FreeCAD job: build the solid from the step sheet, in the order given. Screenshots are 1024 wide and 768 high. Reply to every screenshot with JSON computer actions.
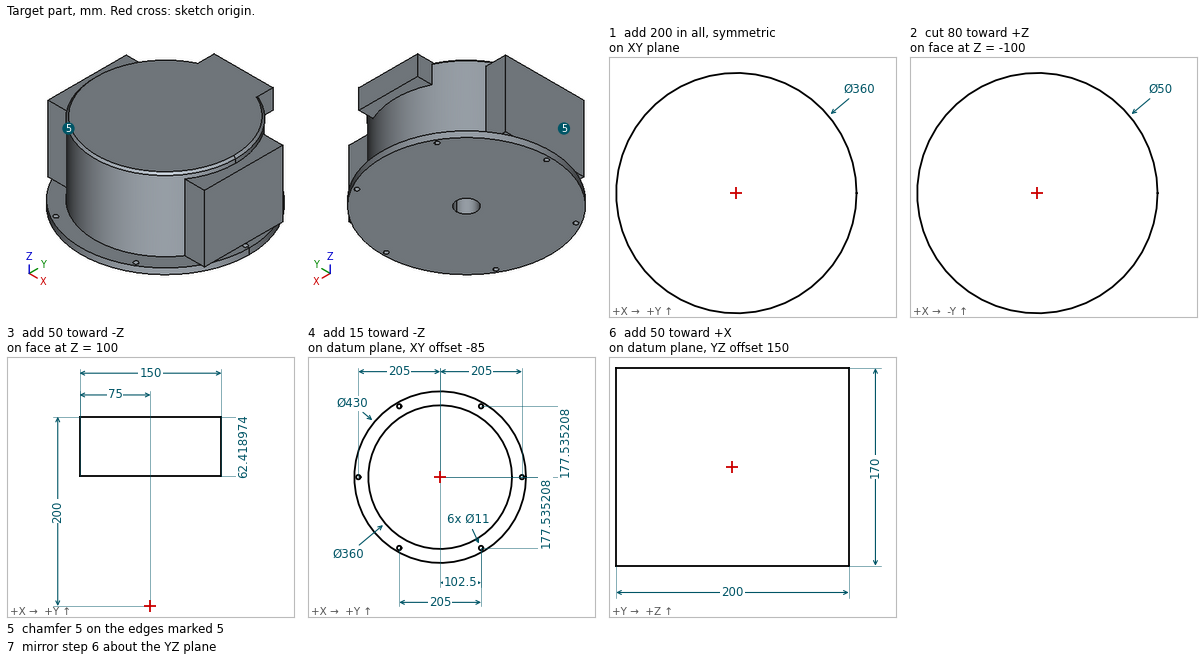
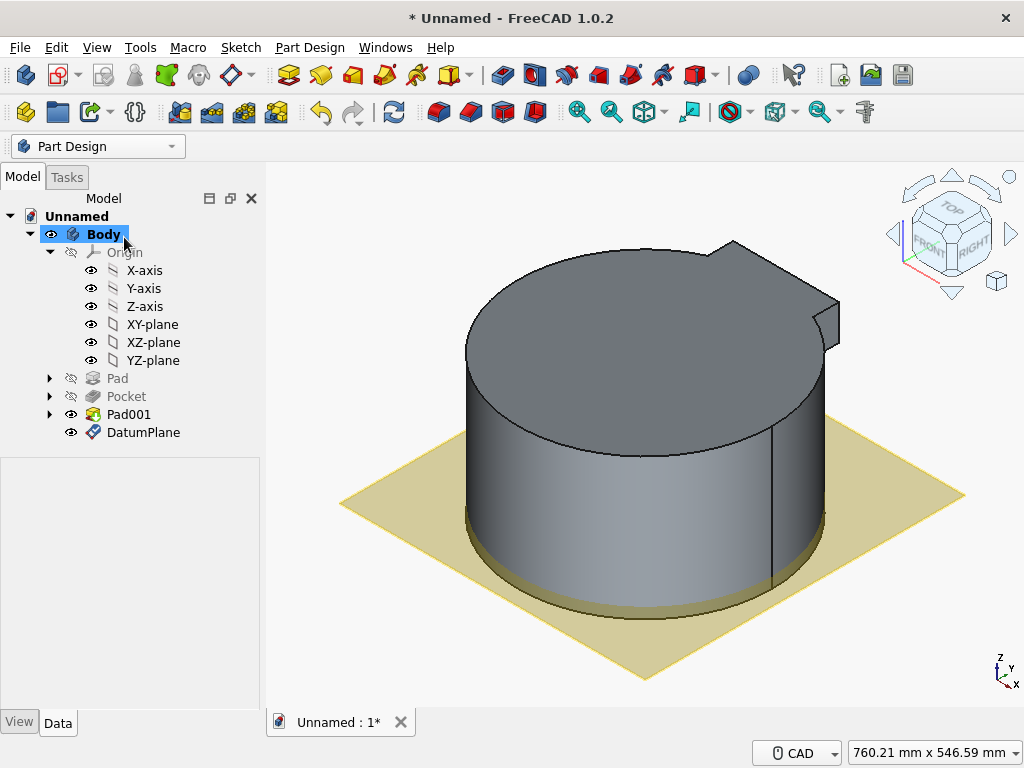
{"action": "left_click", "coordinate": [116, 432]}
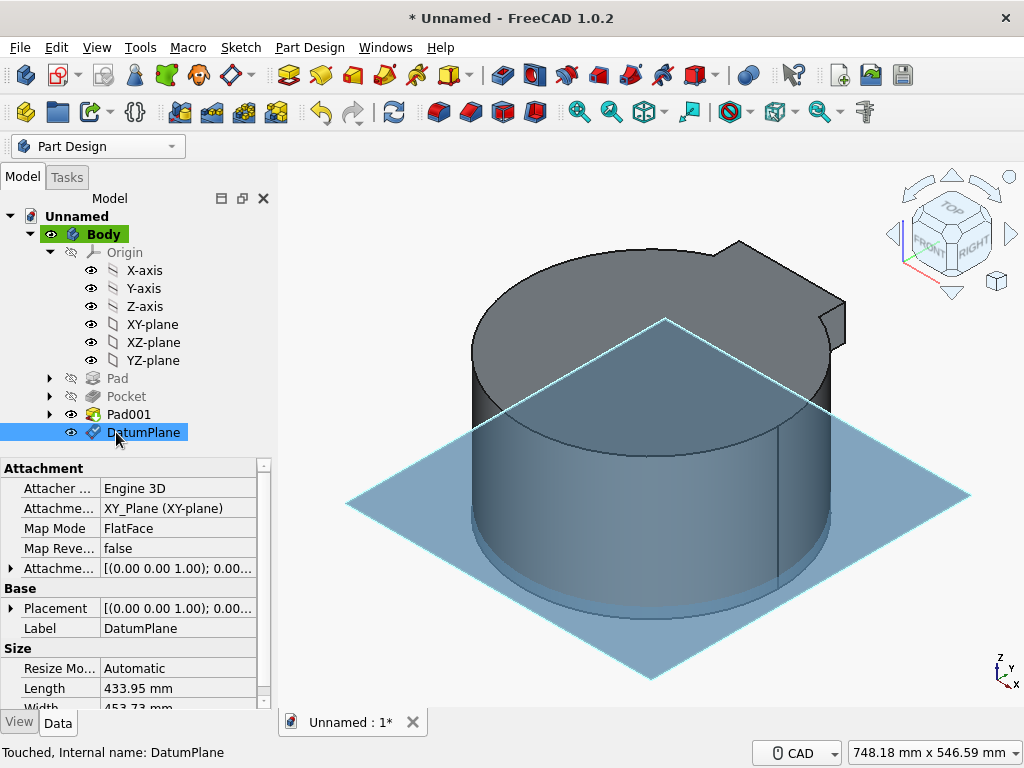
{"action": "left_click", "coordinate": [58, 76]}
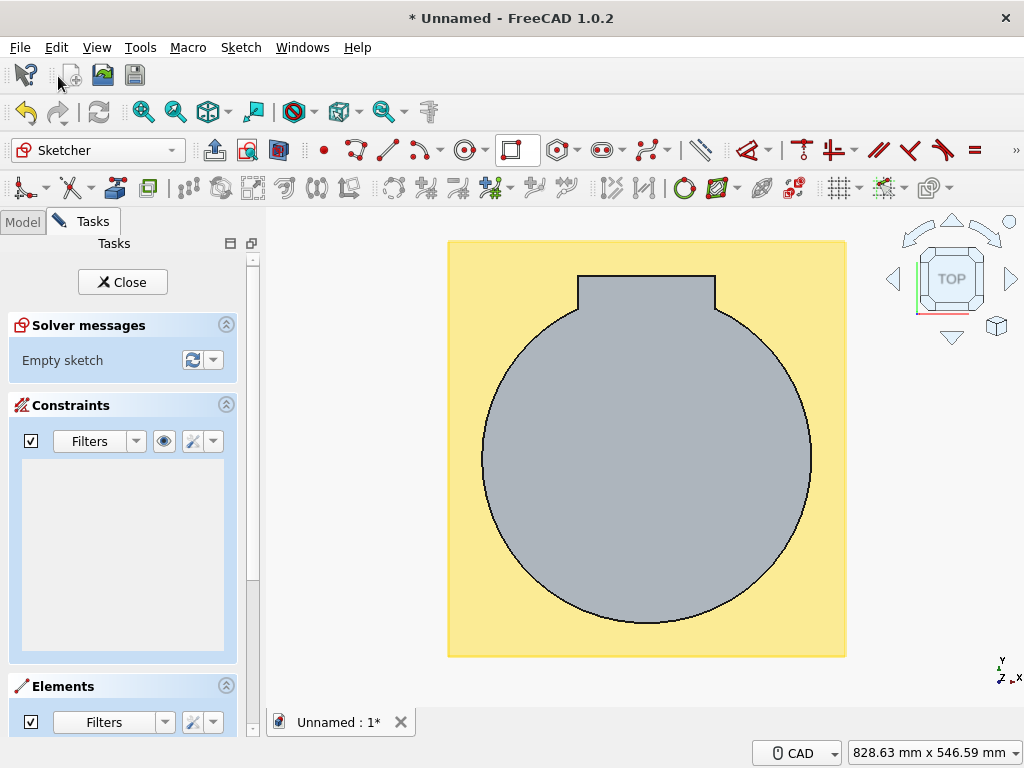
{"action": "left_click", "coordinate": [280, 150]}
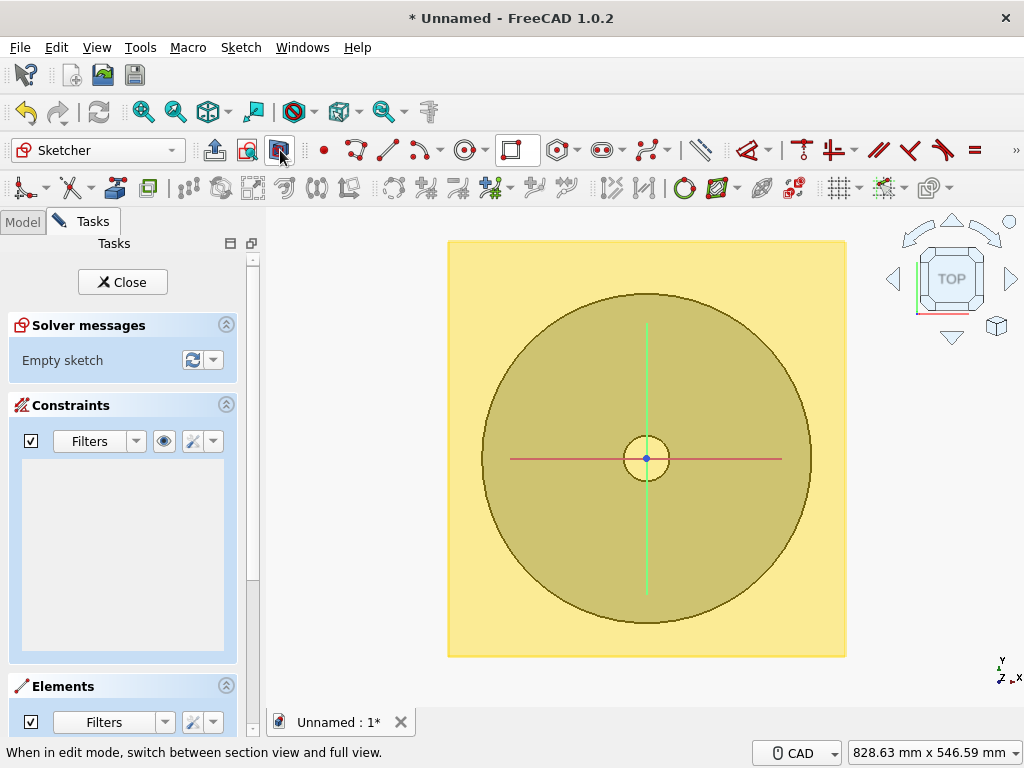
{"action": "scroll", "coordinate": [294, 450], "scroll_direction": "down", "scroll_amount": 1}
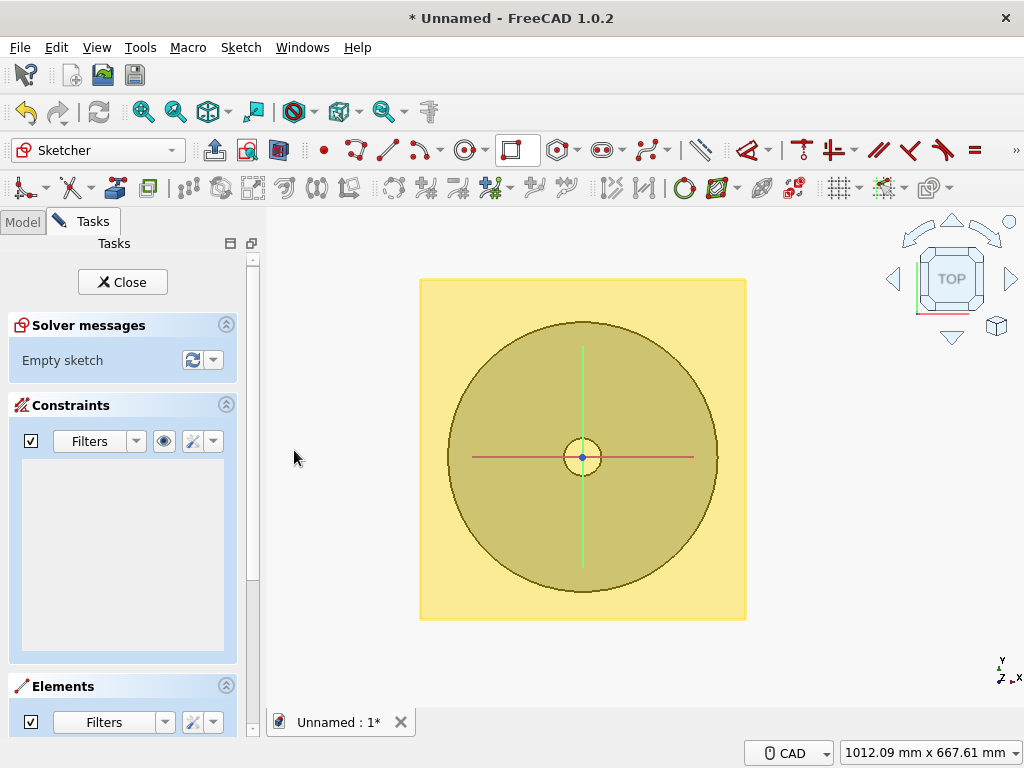
{"action": "key", "text": "g c"}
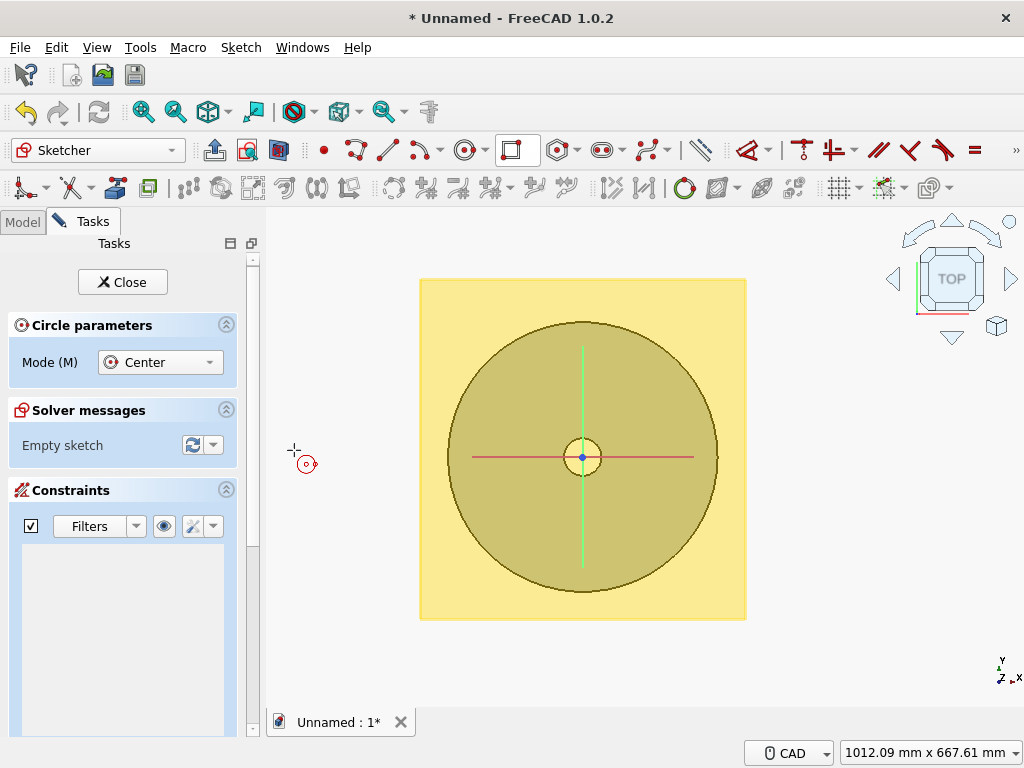
{"action": "left_click", "coordinate": [583, 457]}
{"action": "mouse_move", "coordinate": [697, 343]}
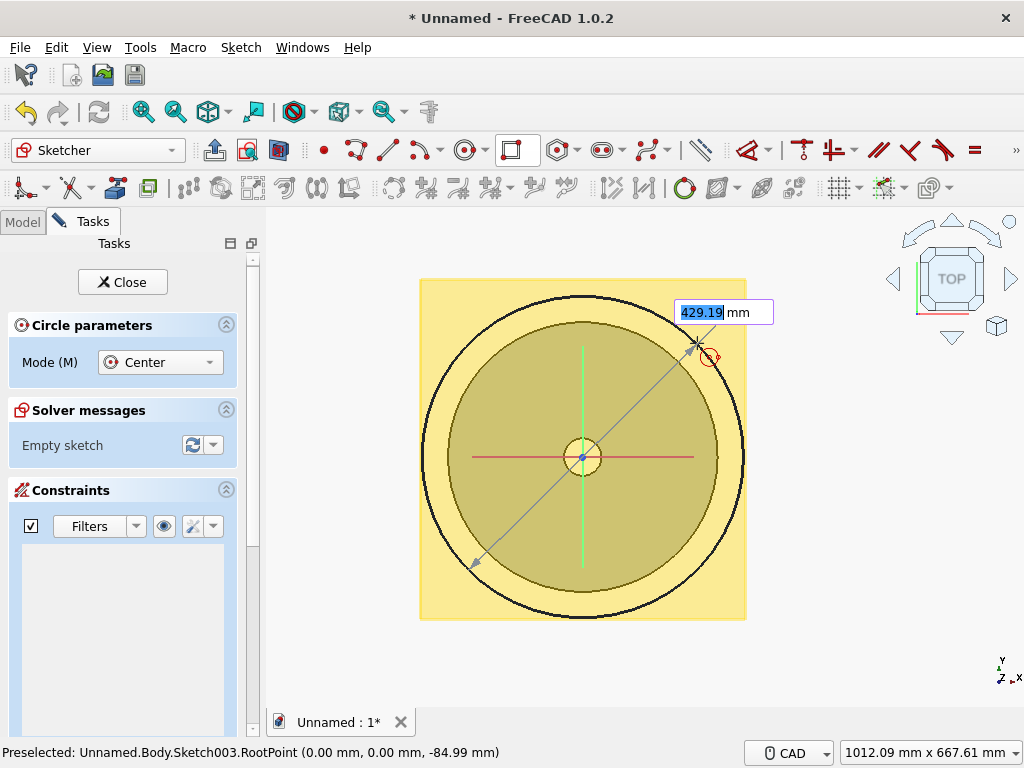
{"action": "type", "text": "430"}
{"action": "key", "text": "Return"}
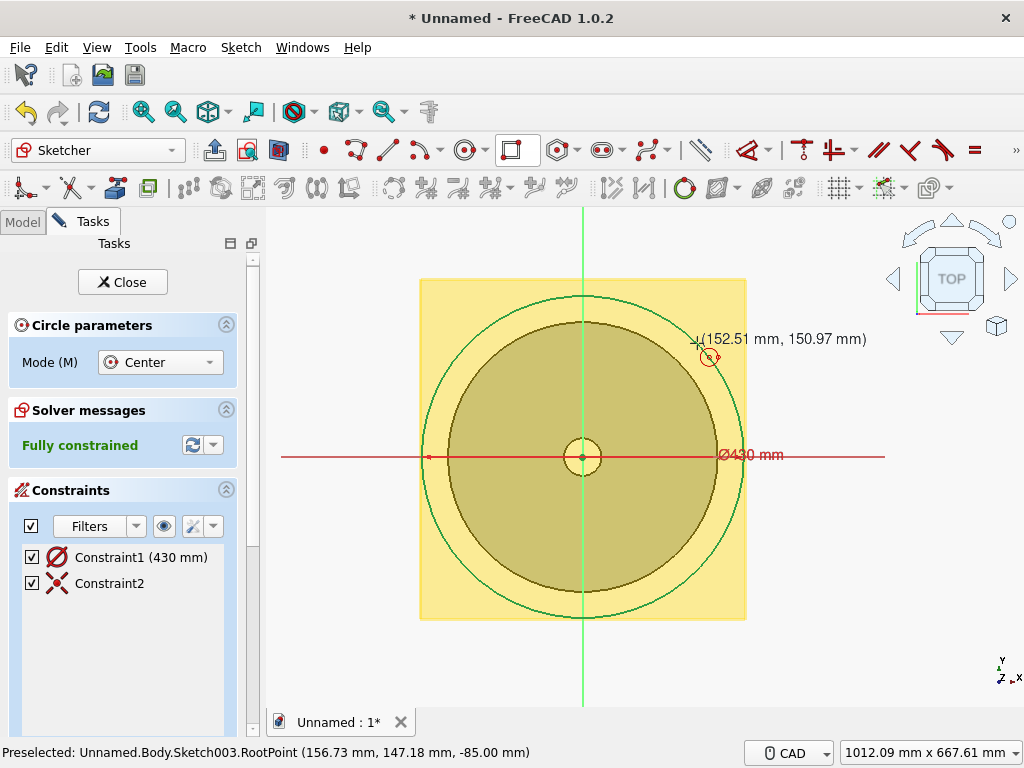
{"action": "scroll", "coordinate": [660, 590], "scroll_direction": "up", "scroll_amount": 9}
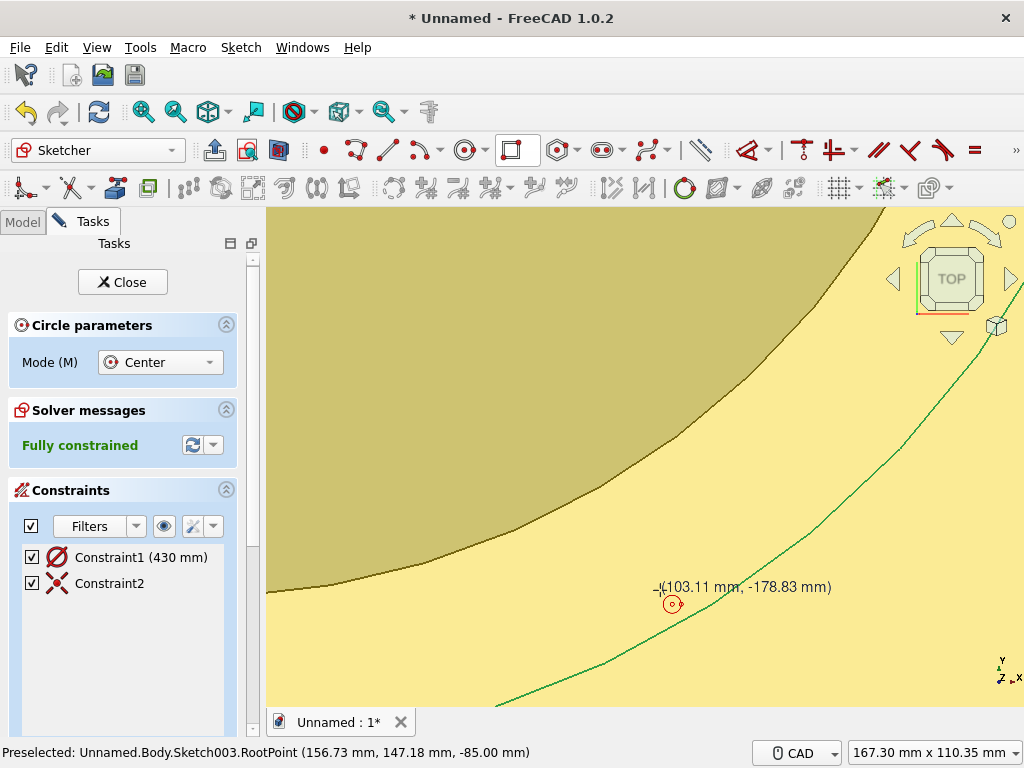
{"action": "left_click", "coordinate": [655, 586]}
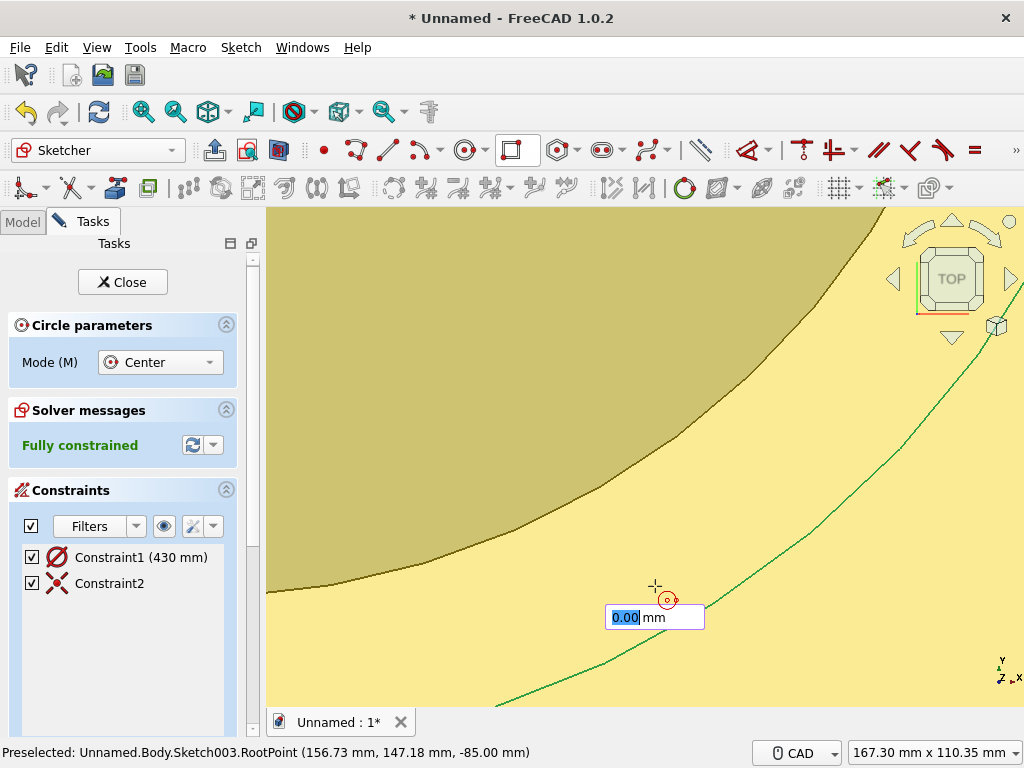
{"action": "scroll", "coordinate": [653, 591], "scroll_direction": "down", "scroll_amount": 9}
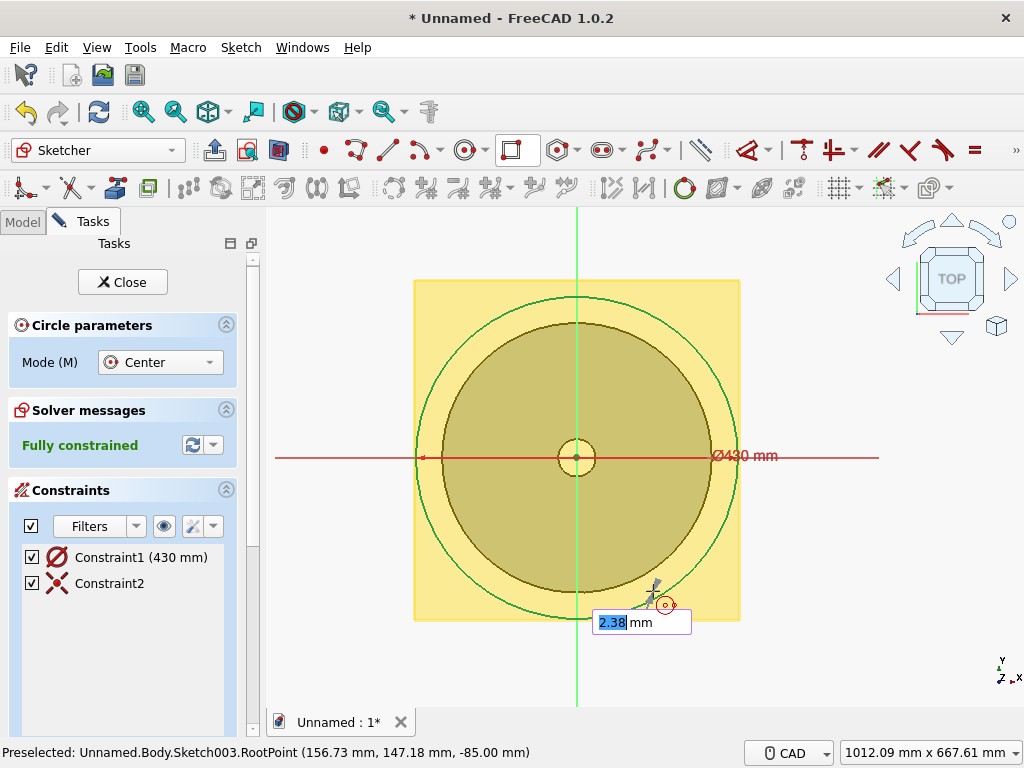
{"action": "scroll", "coordinate": [657, 588], "scroll_direction": "up", "scroll_amount": 4}
{"action": "mouse_move", "coordinate": [655, 587]}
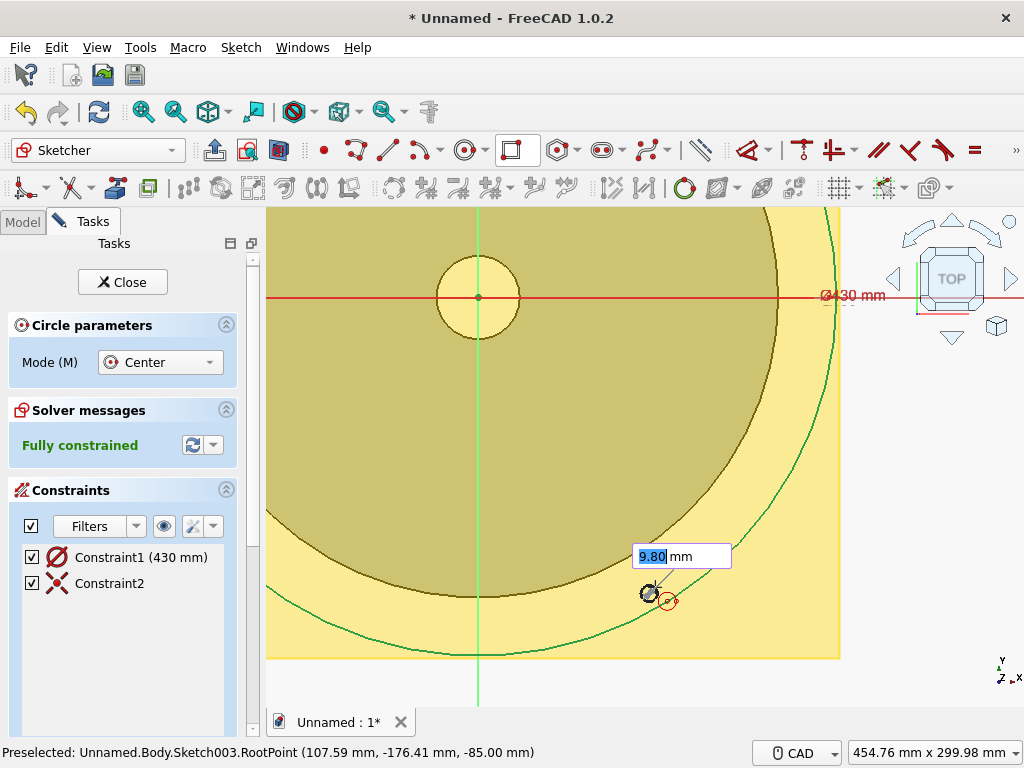
{"action": "type", "text": "11"}
{"action": "key", "text": "Return"}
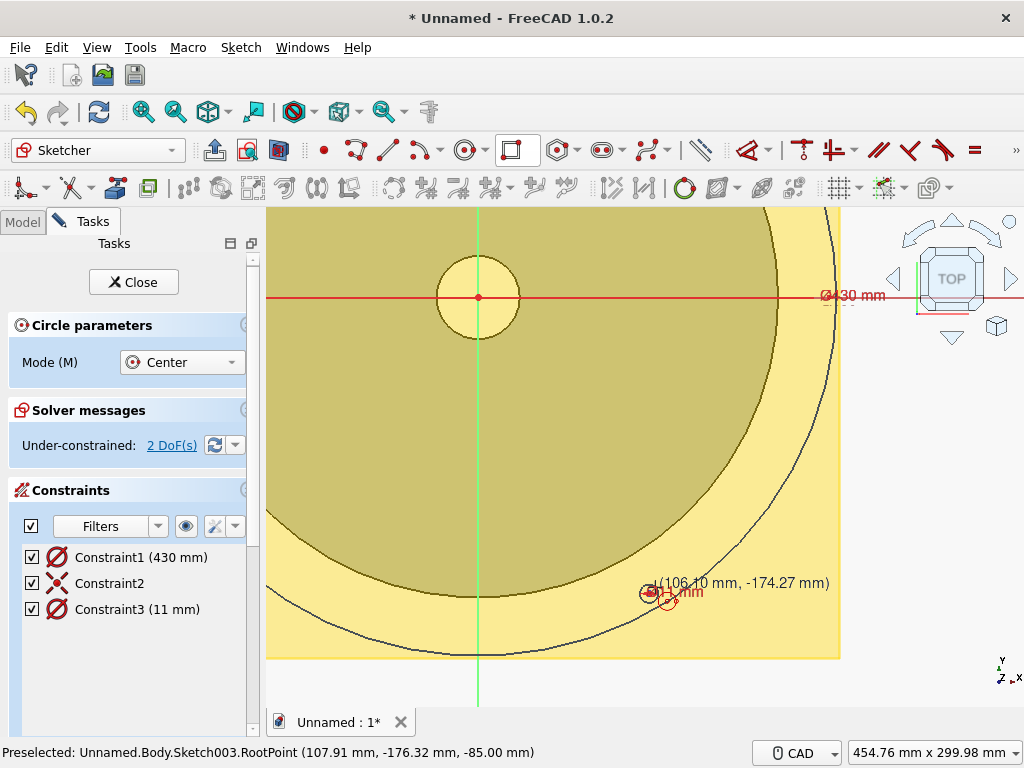
{"action": "scroll", "coordinate": [307, 593], "scroll_direction": "up", "scroll_amount": 5}